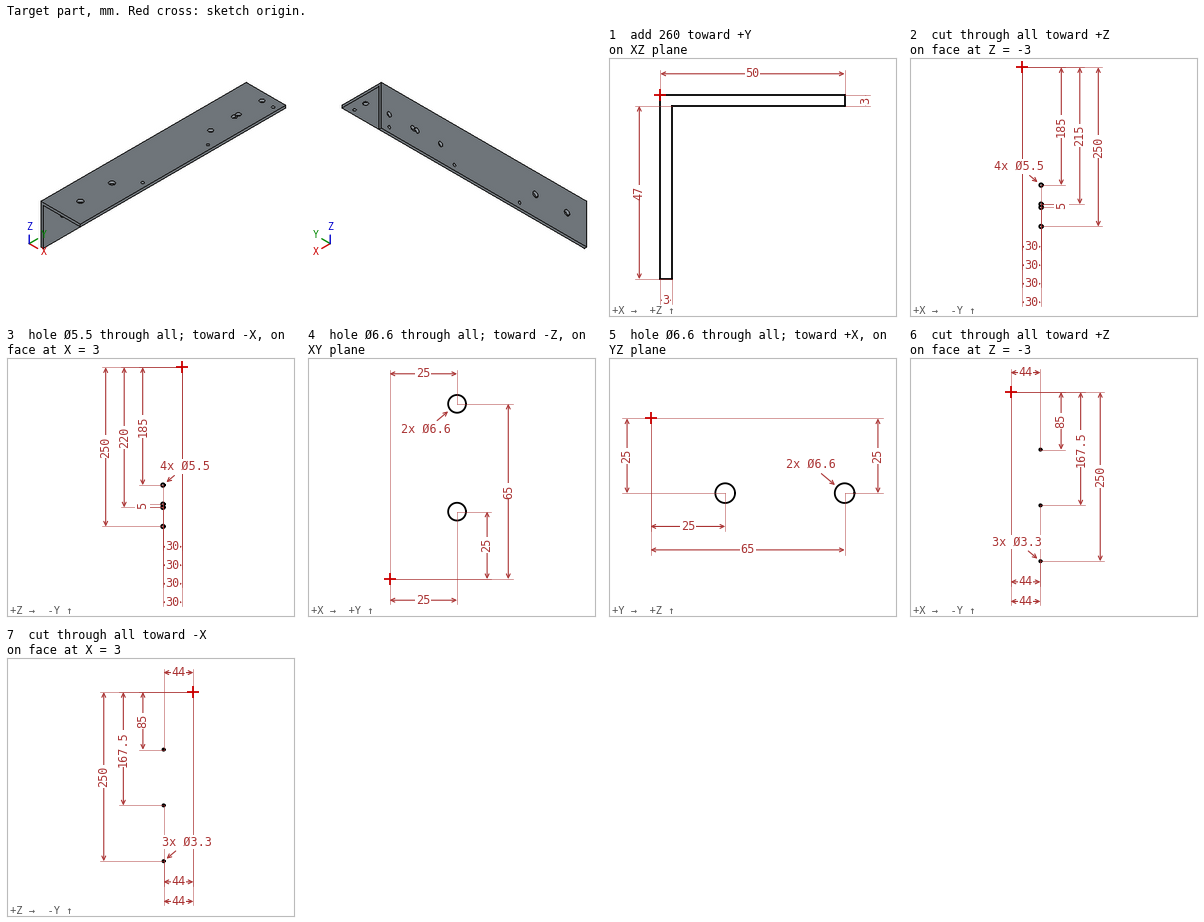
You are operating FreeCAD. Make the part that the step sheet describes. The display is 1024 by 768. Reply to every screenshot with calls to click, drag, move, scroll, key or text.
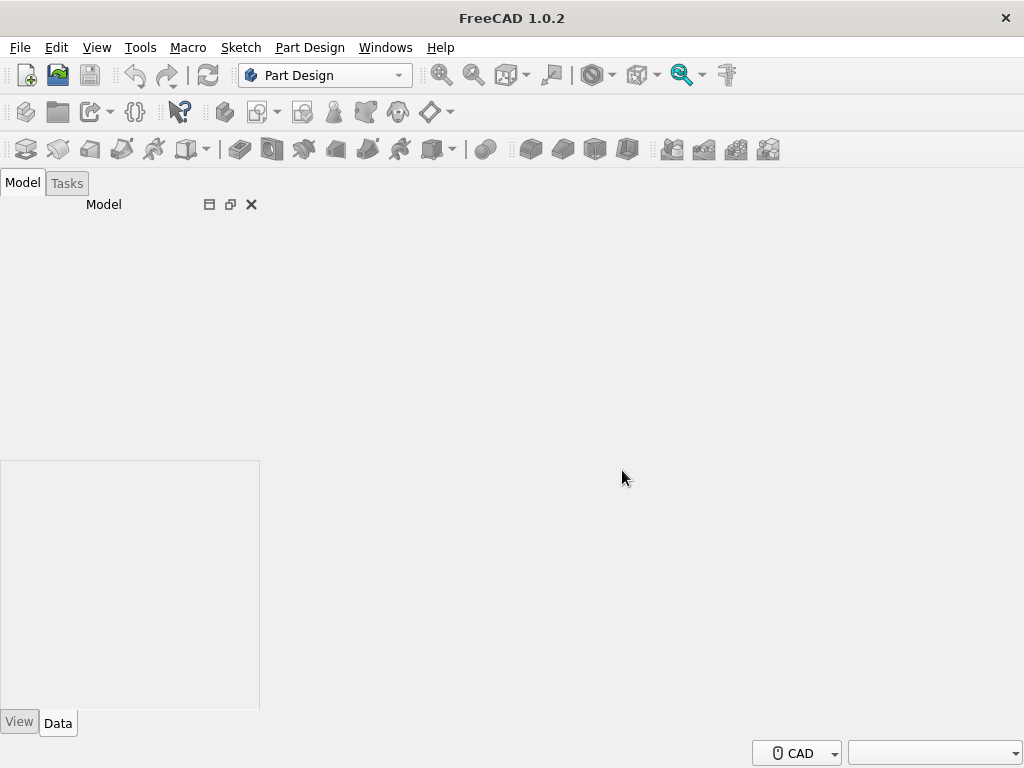
key(ctrl+n)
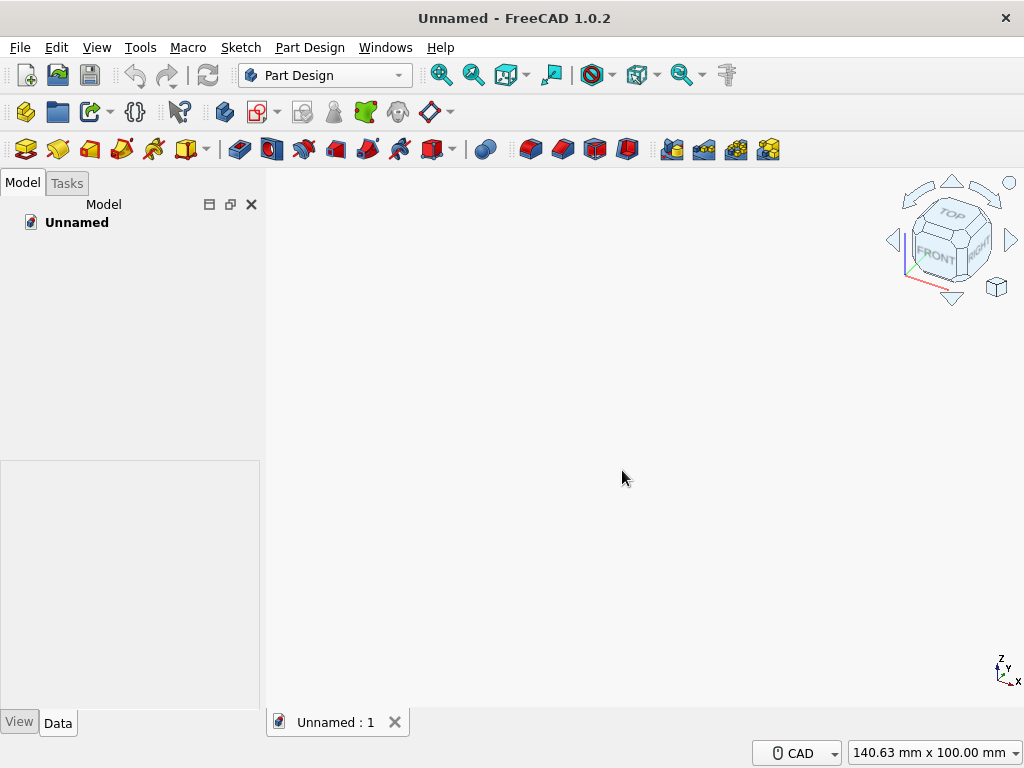
click(258, 112)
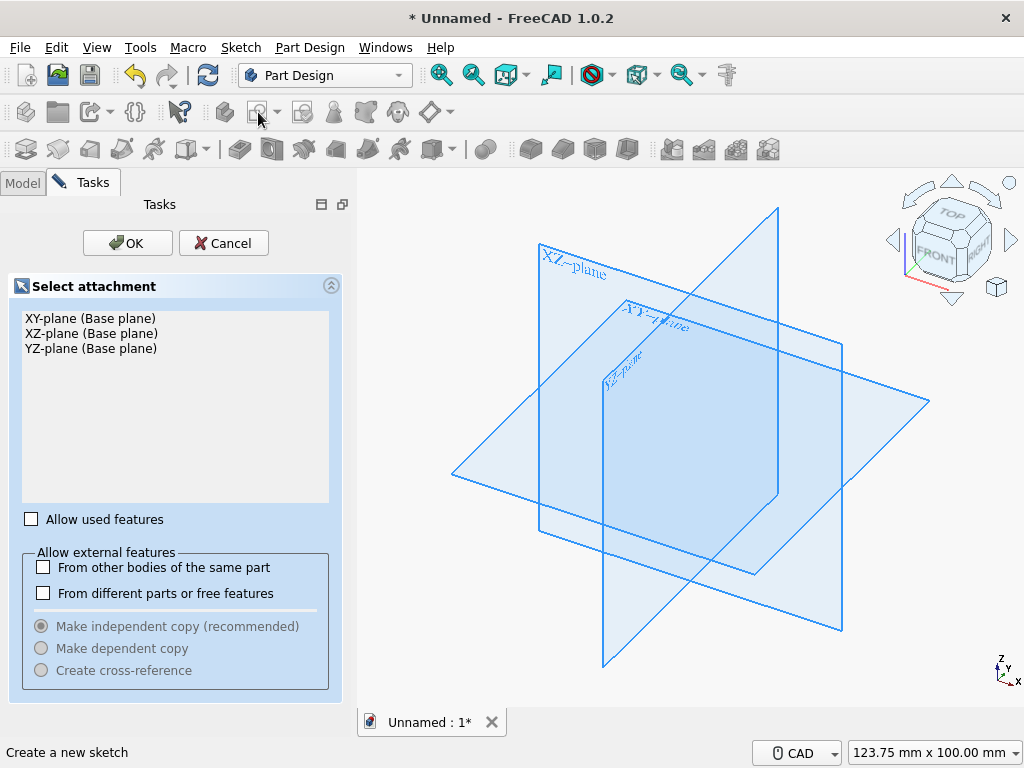
click(82, 334)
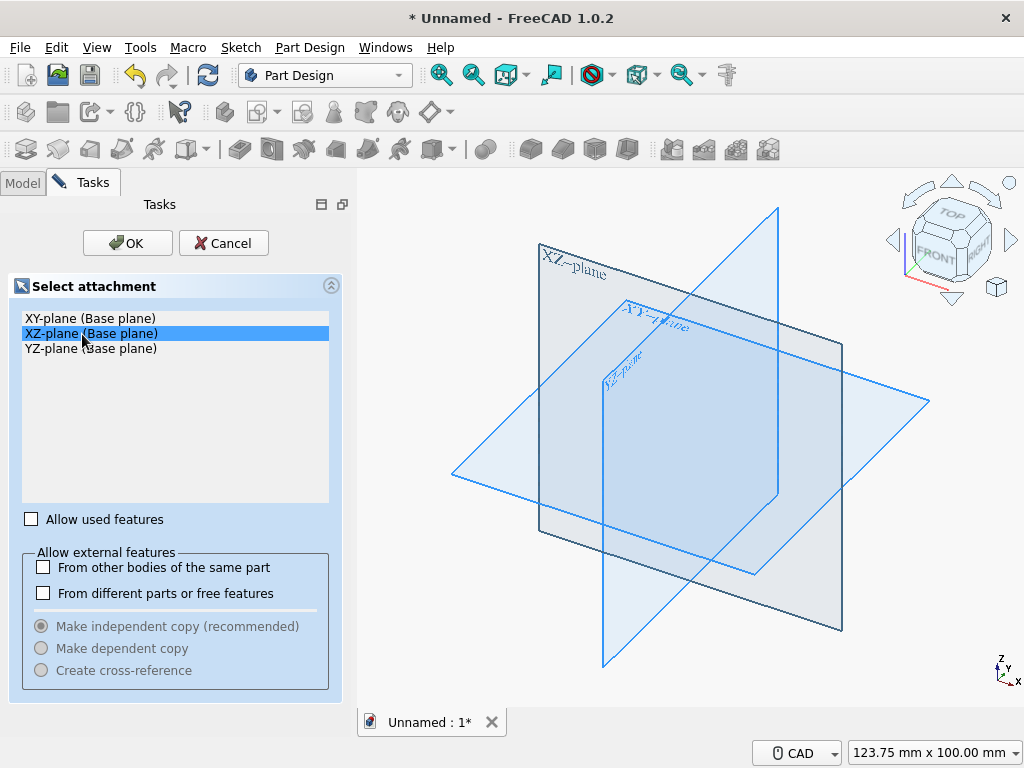
click(128, 243)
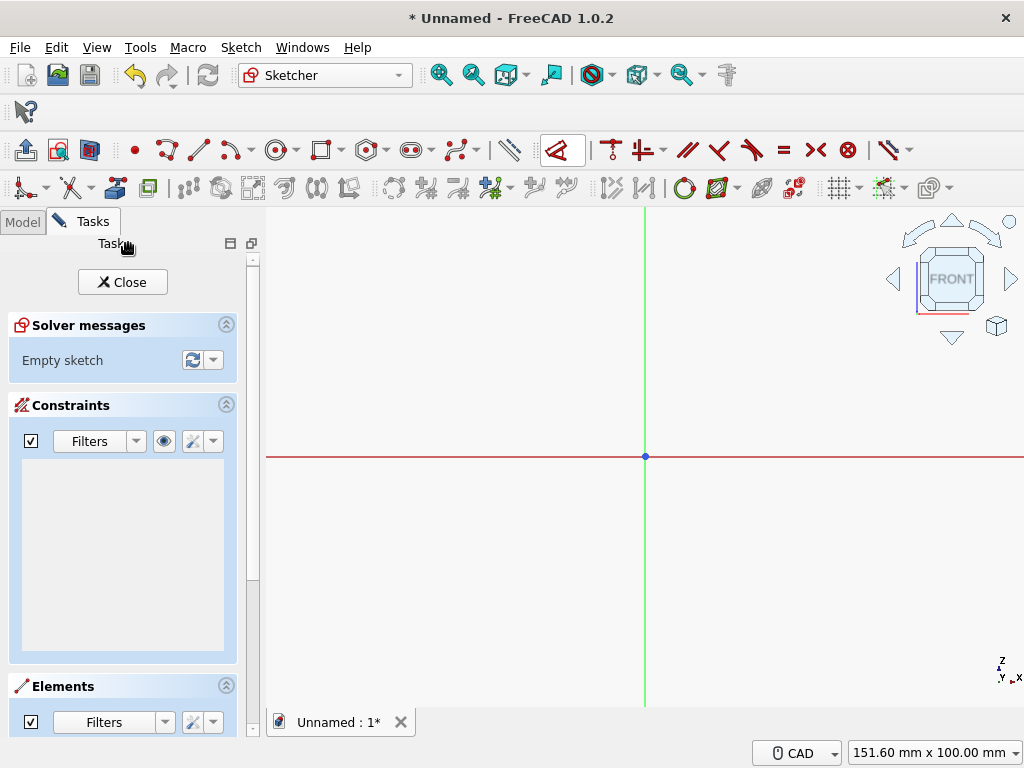
scroll(294, 235, down, 1)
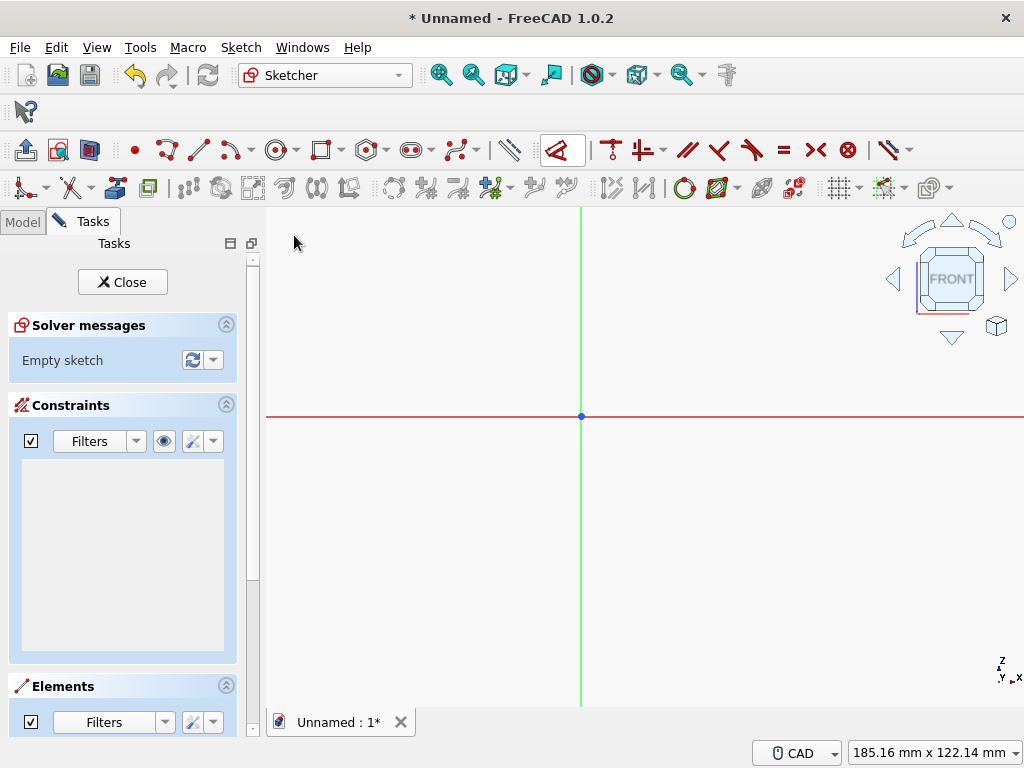
scroll(859, 645, up, 2)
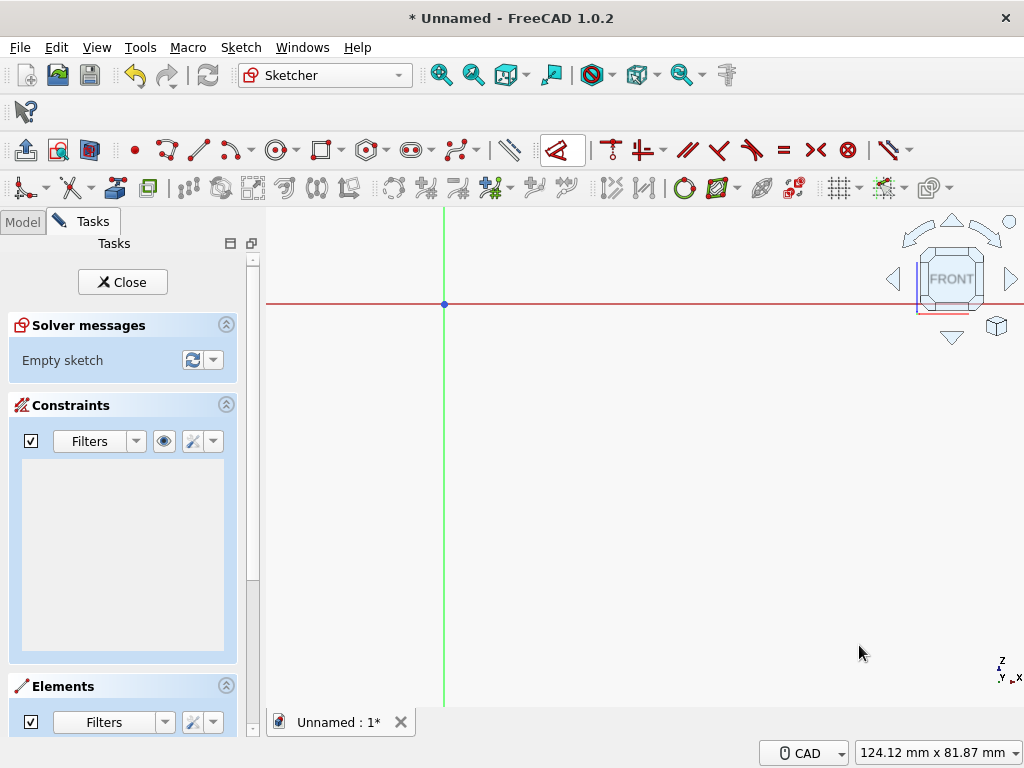
key(g)
key(m)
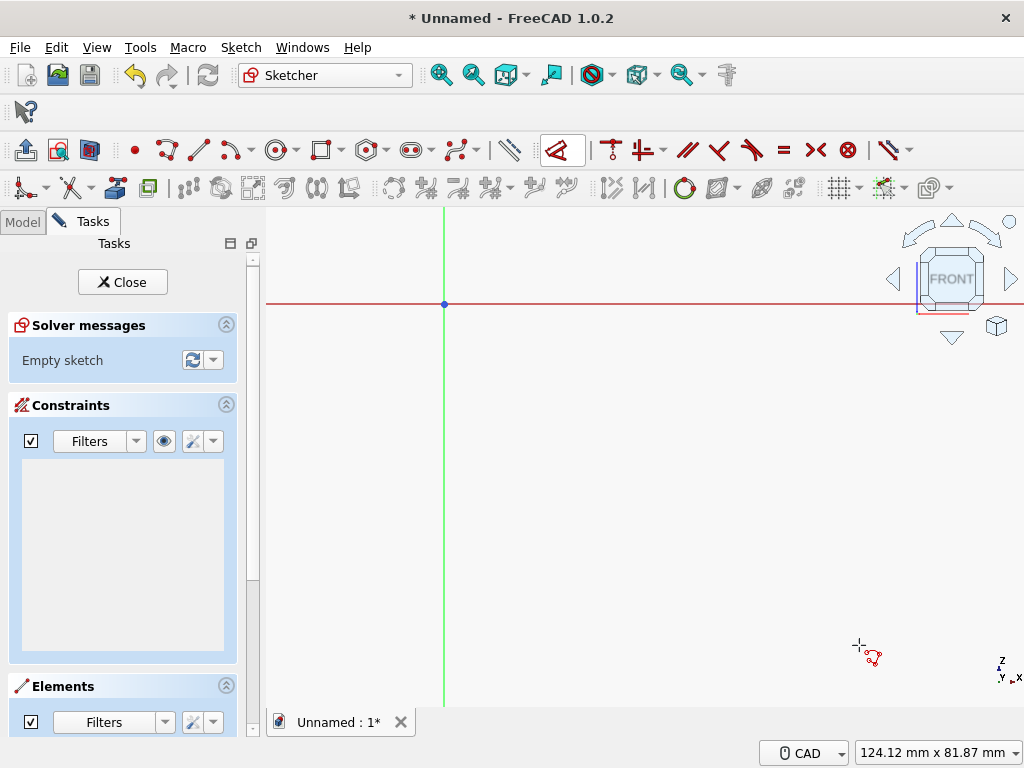
click(444, 304)
click(750, 313)
click(750, 322)
click(463, 322)
click(463, 609)
click(453, 609)
click(444, 304)
key(Escape)
key(Escape)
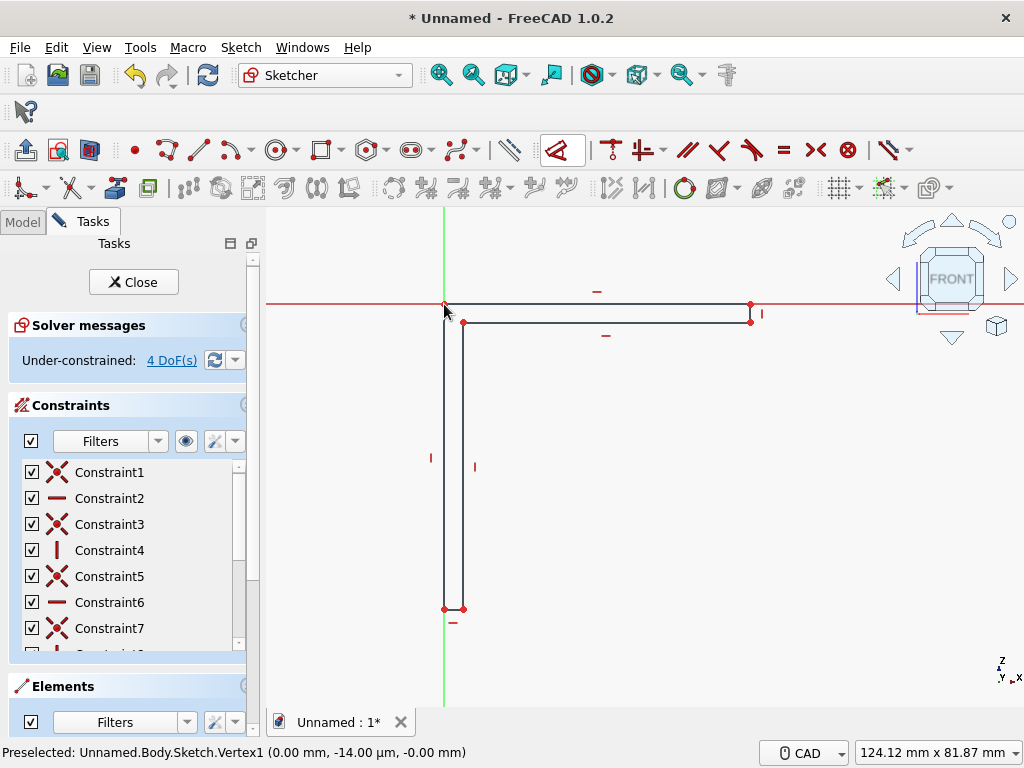
scroll(750, 314, up, 4)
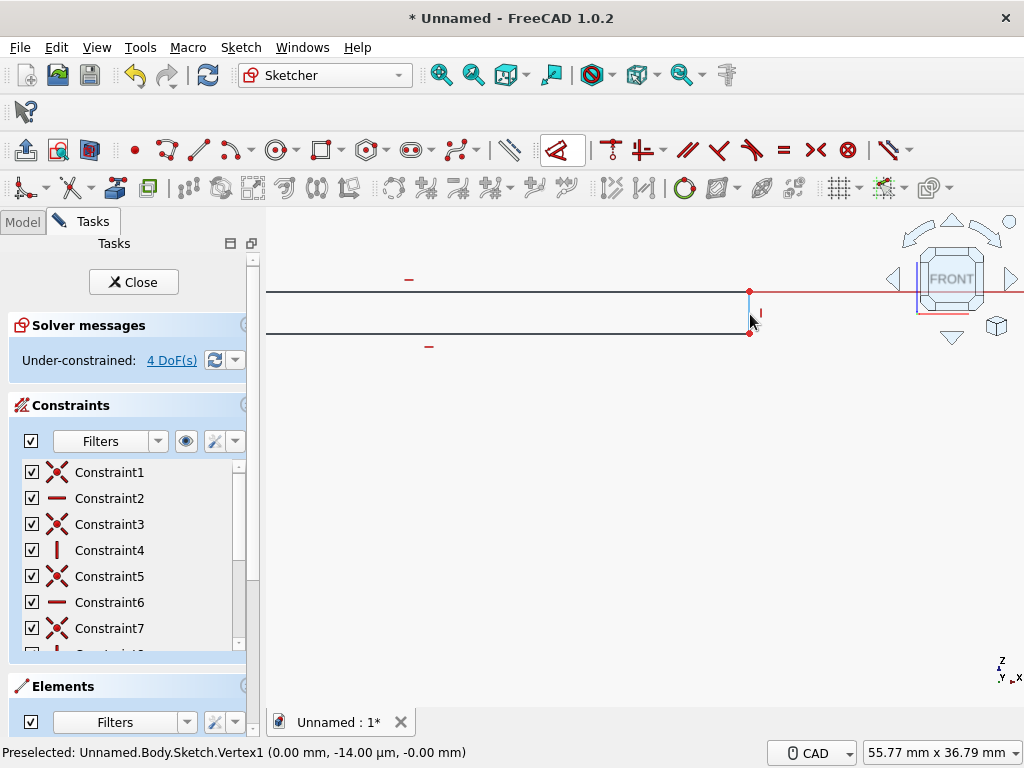
click(749, 313)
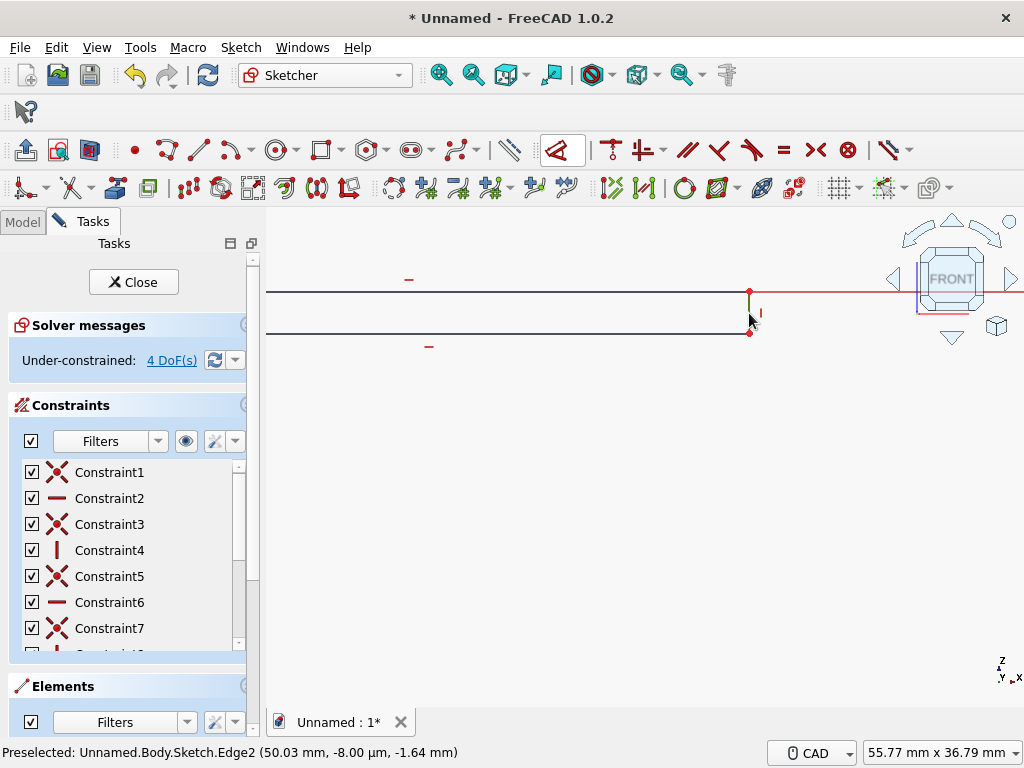
key(i)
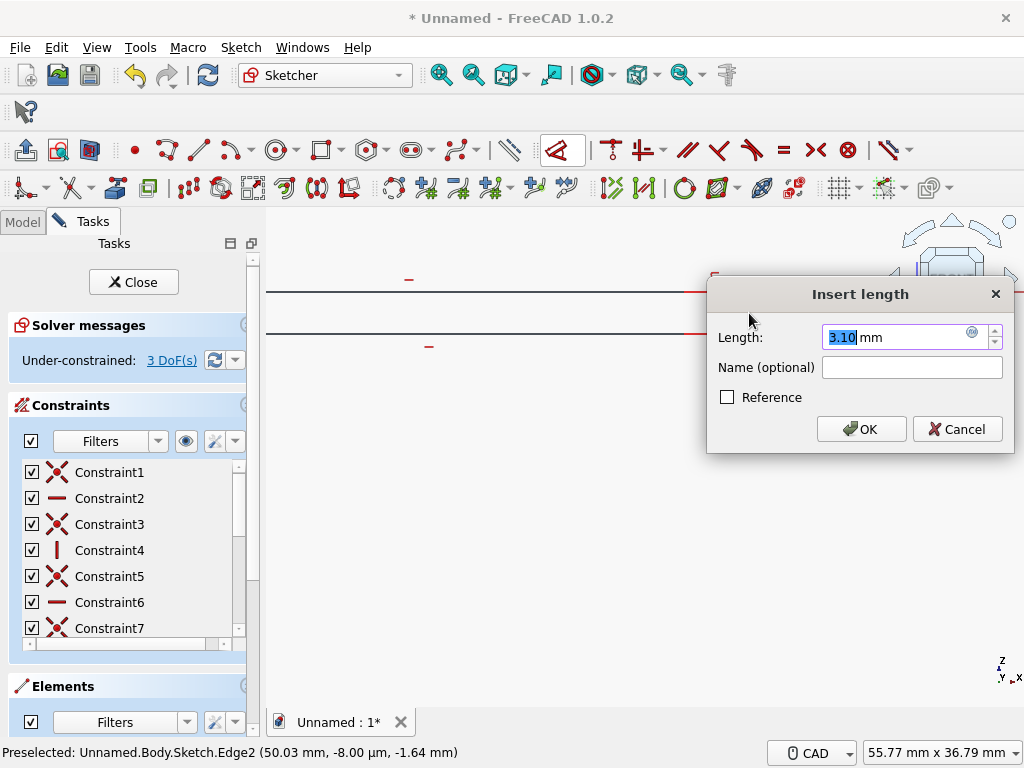
text(3)
key(Return)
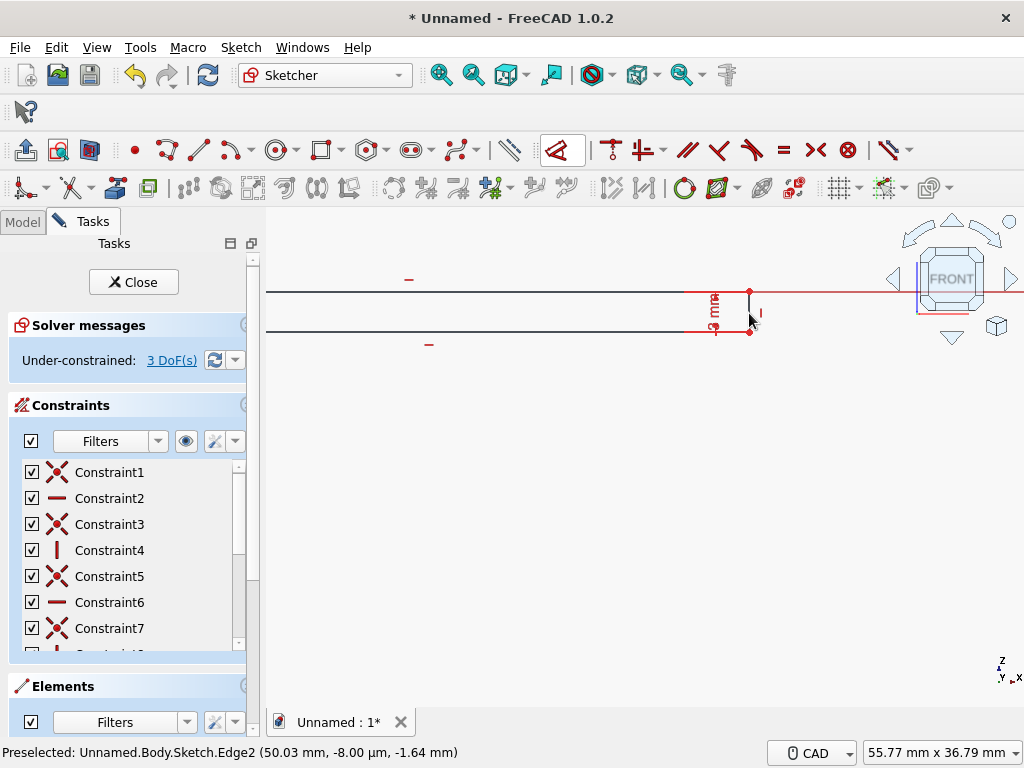
scroll(713, 315, down, 4)